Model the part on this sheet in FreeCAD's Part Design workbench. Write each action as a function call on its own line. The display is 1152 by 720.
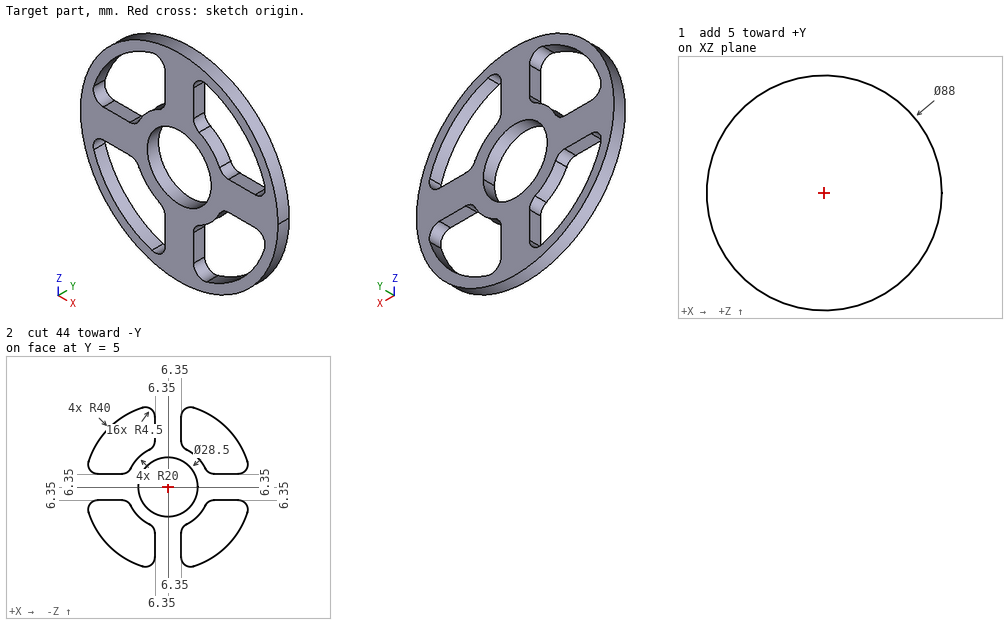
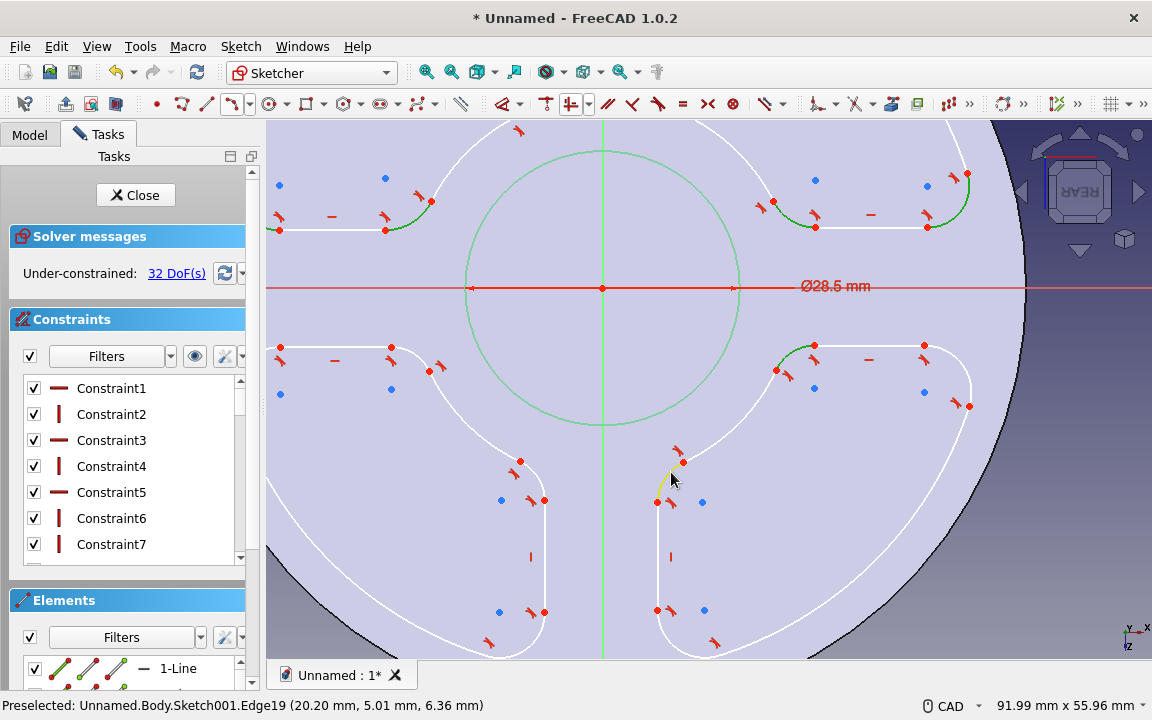
click(671, 471)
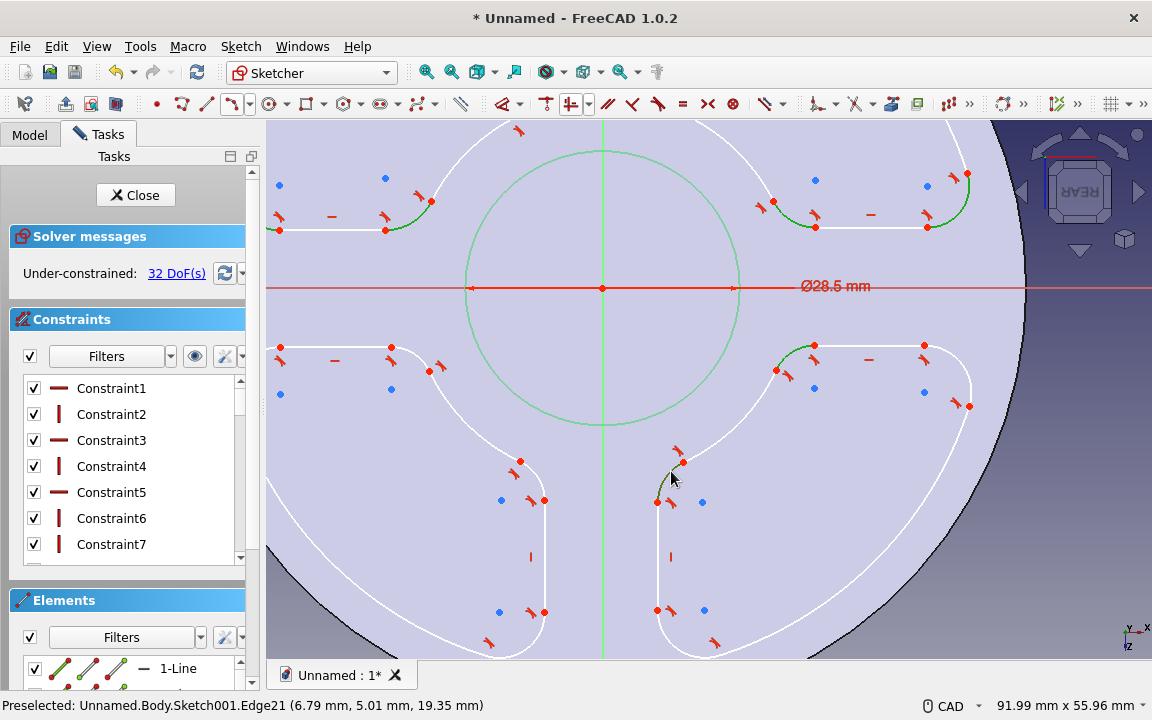
click(661, 628)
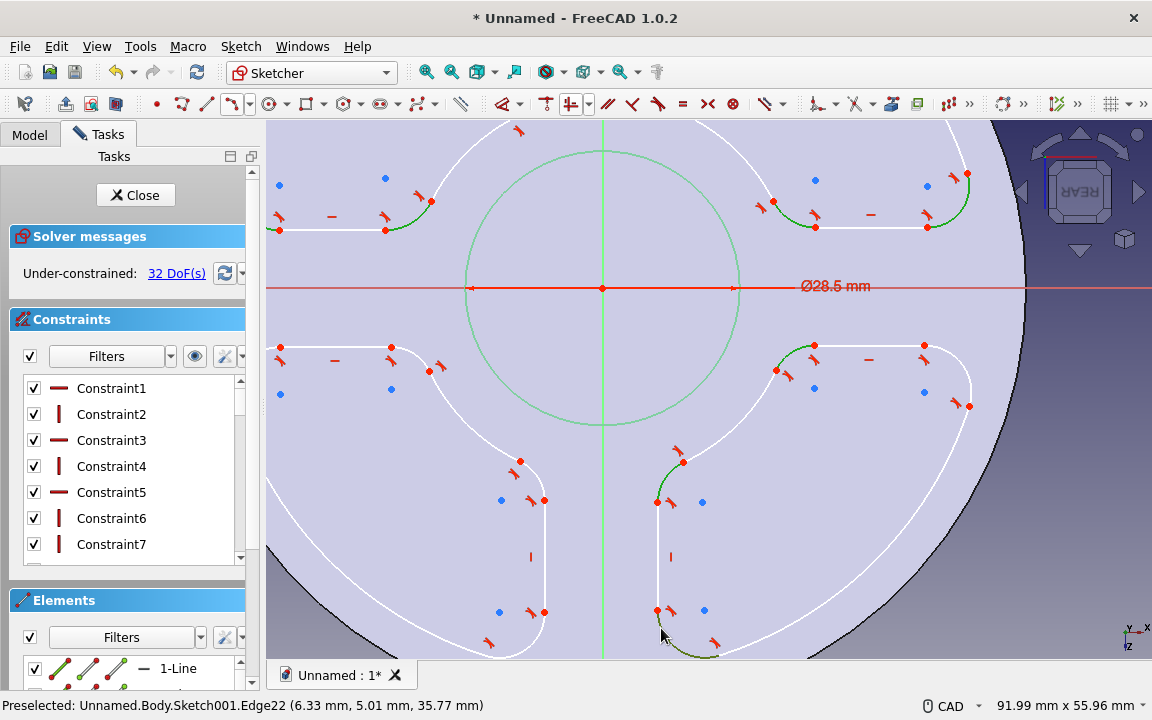
click(970, 381)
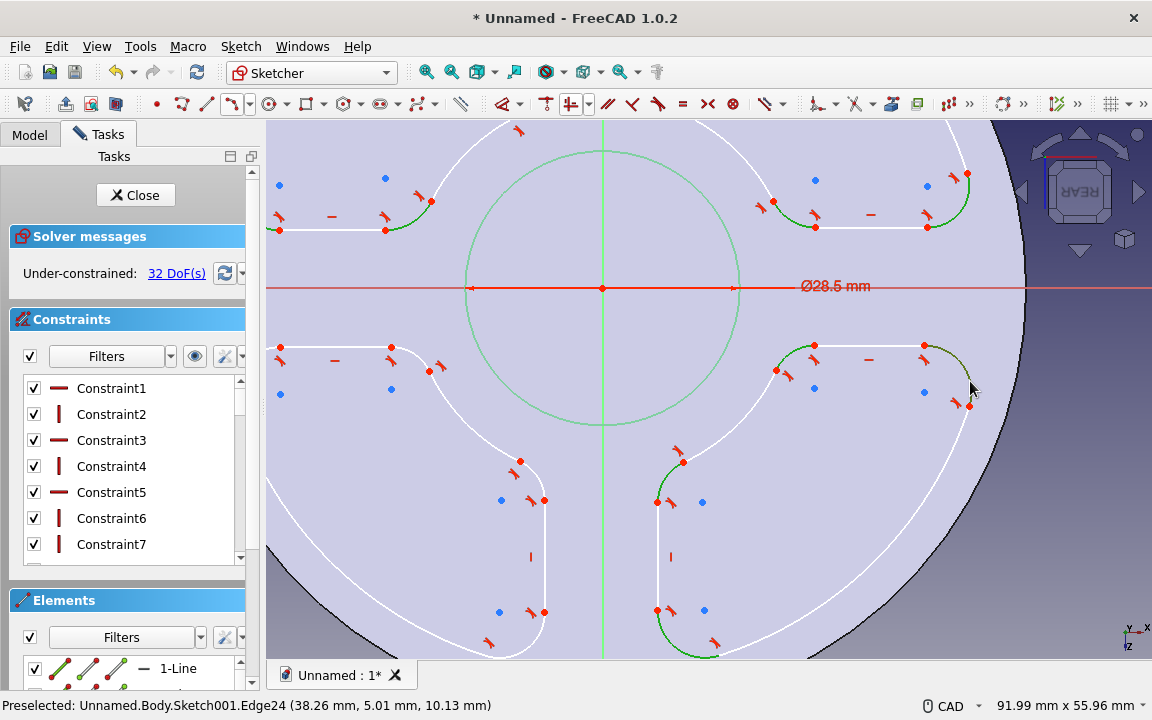
click(542, 486)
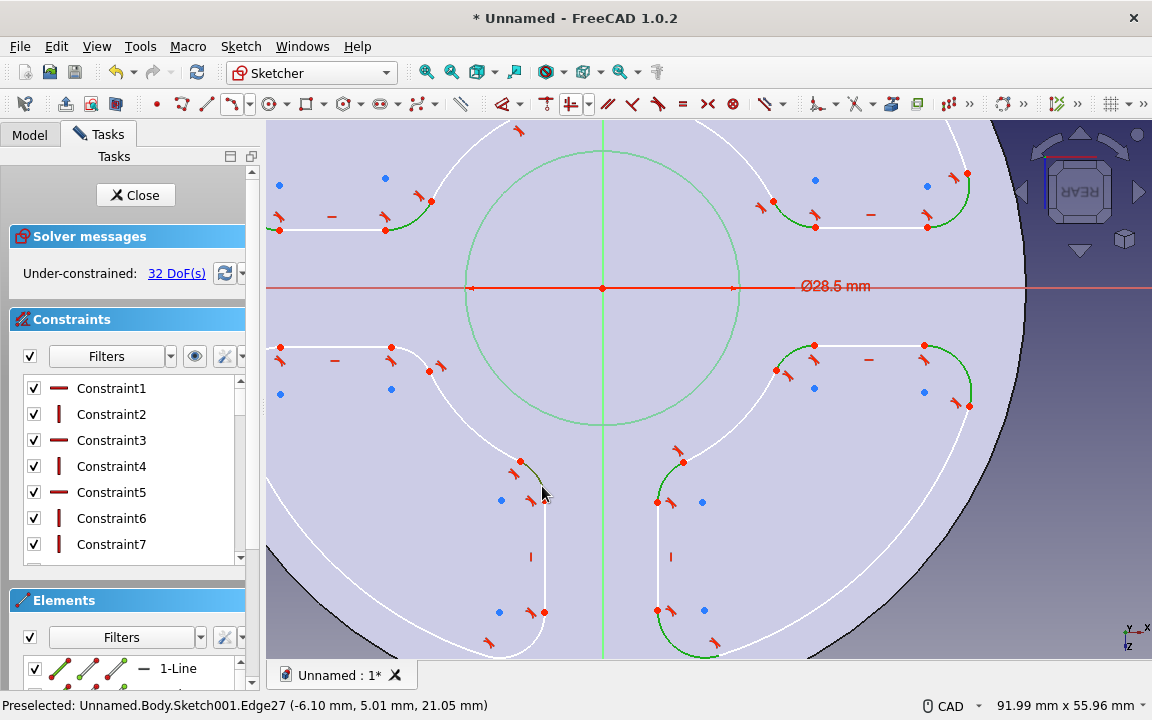
click(421, 360)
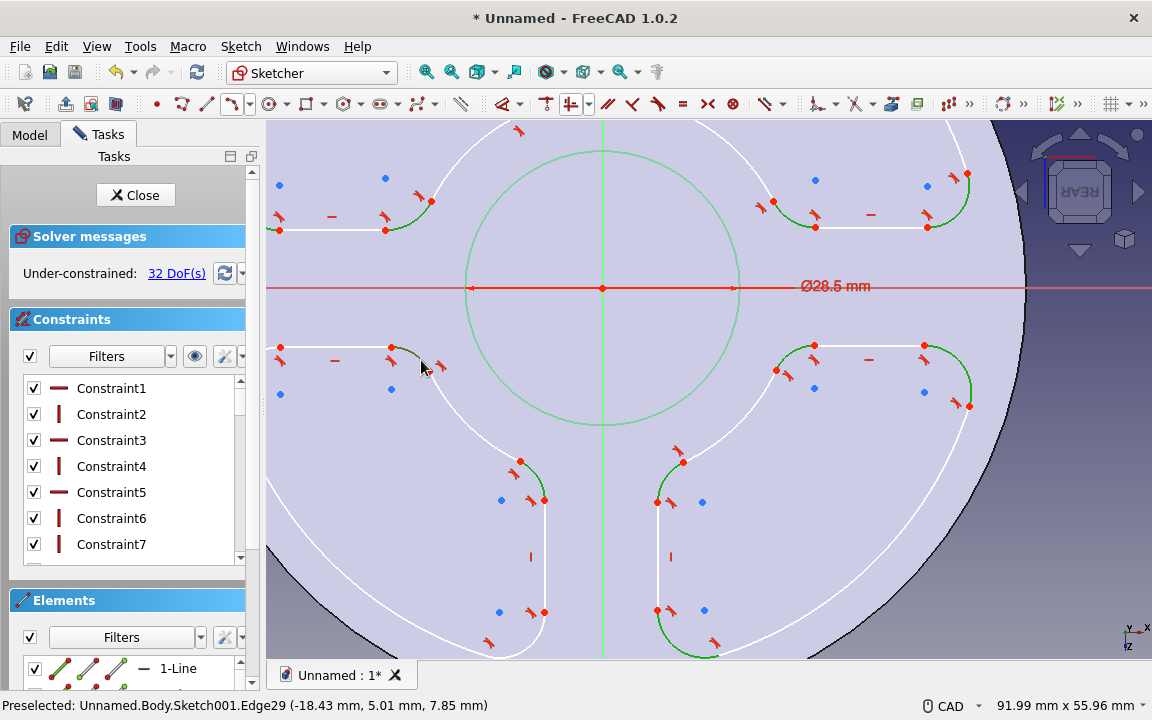
scroll(672, 472, down, 4)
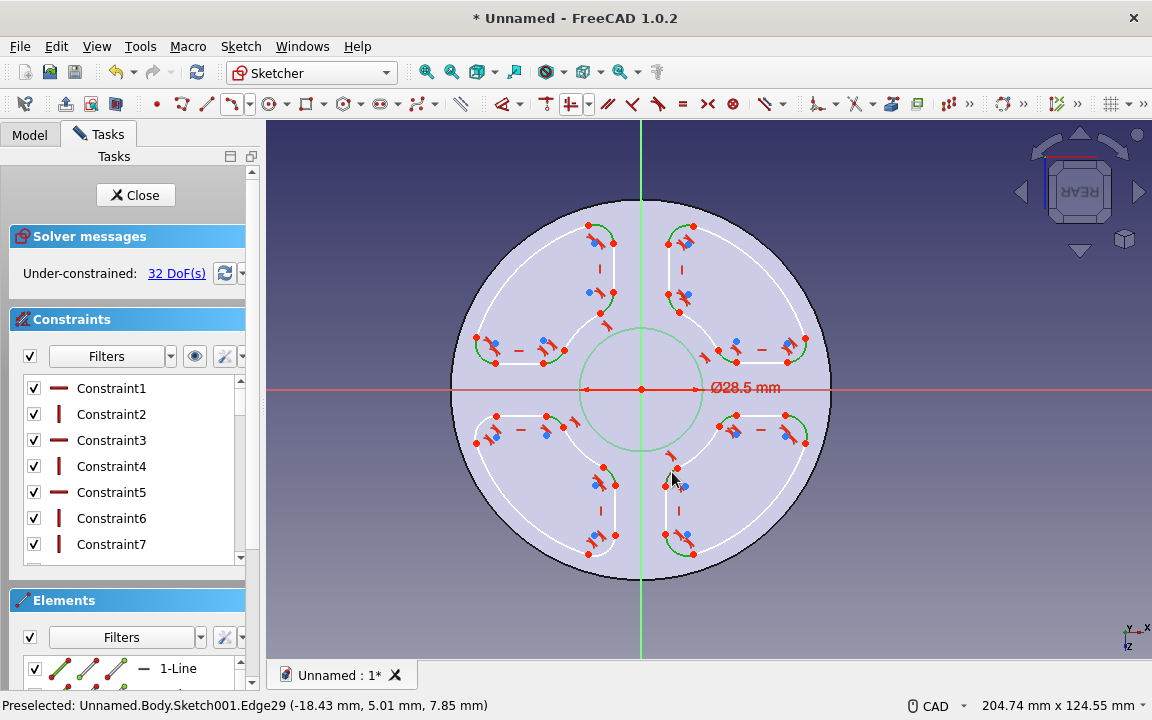
click(485, 420)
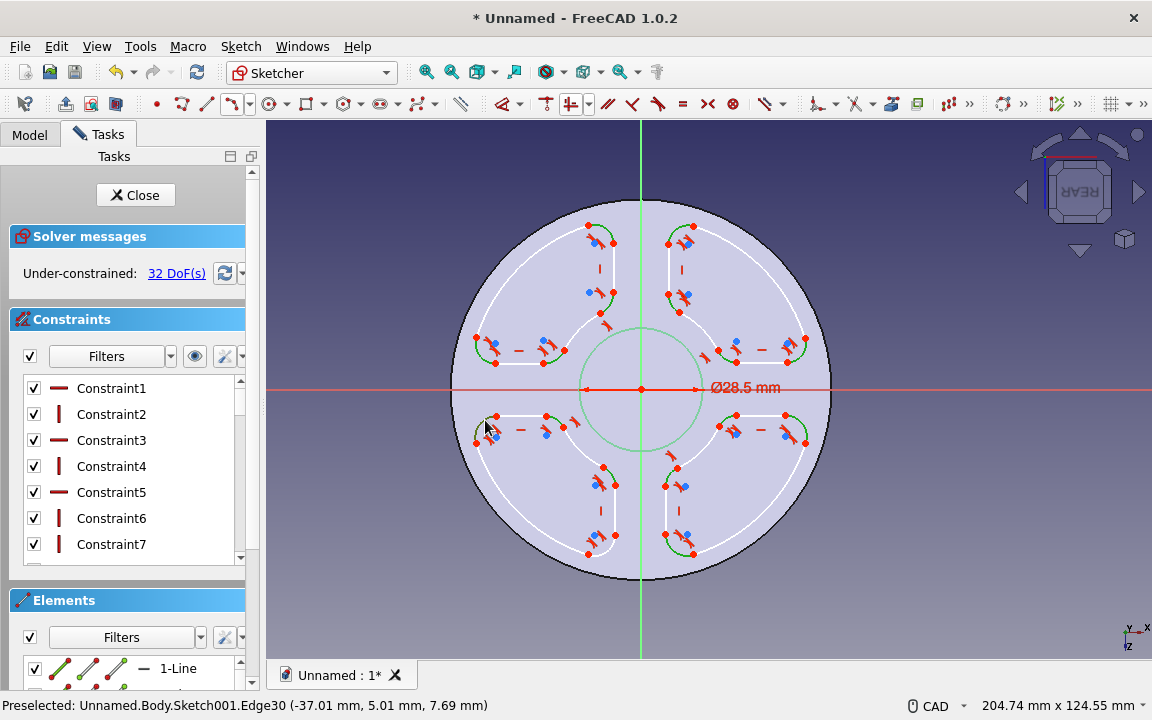
click(600, 555)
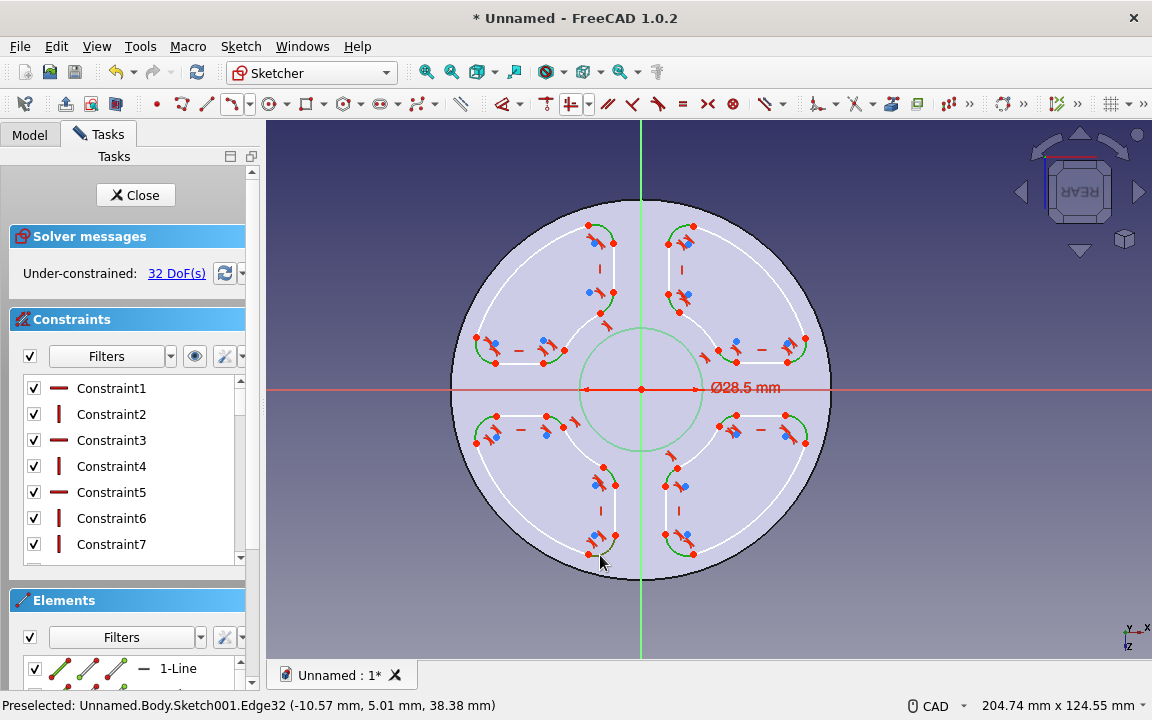
key(e)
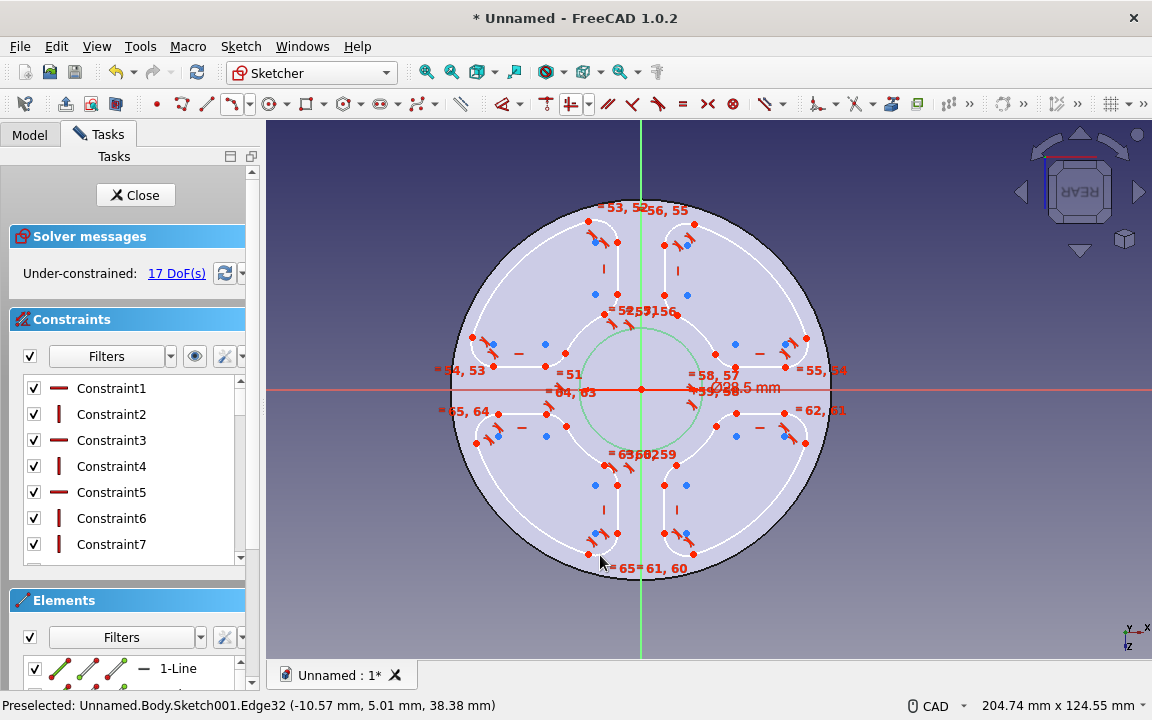
click(542, 243)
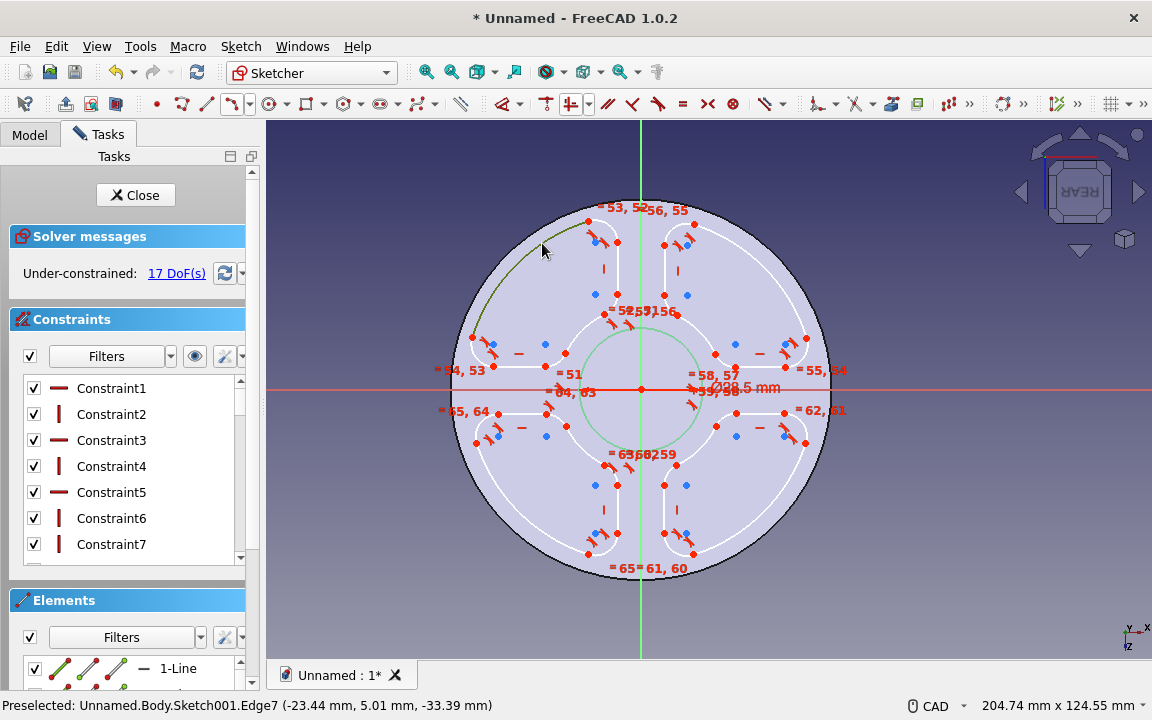
click(785, 293)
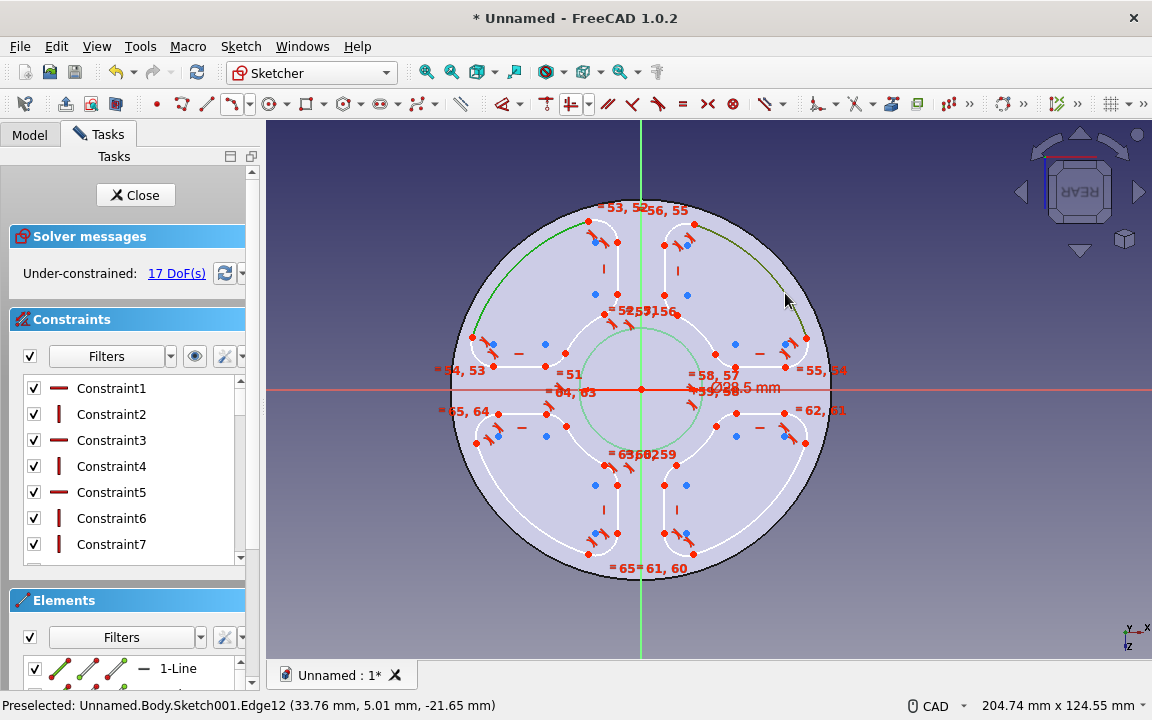
click(738, 533)